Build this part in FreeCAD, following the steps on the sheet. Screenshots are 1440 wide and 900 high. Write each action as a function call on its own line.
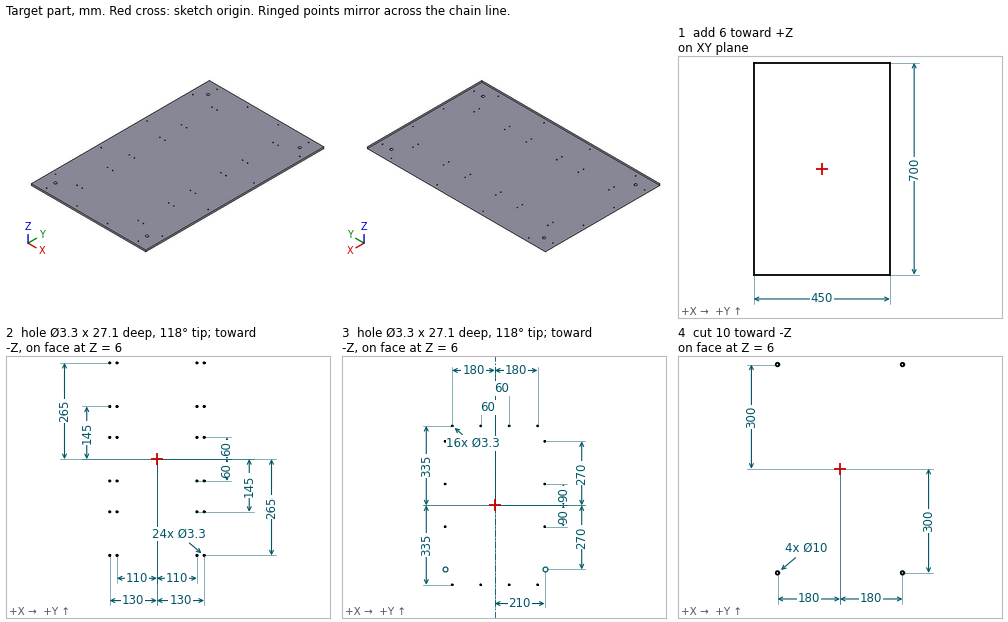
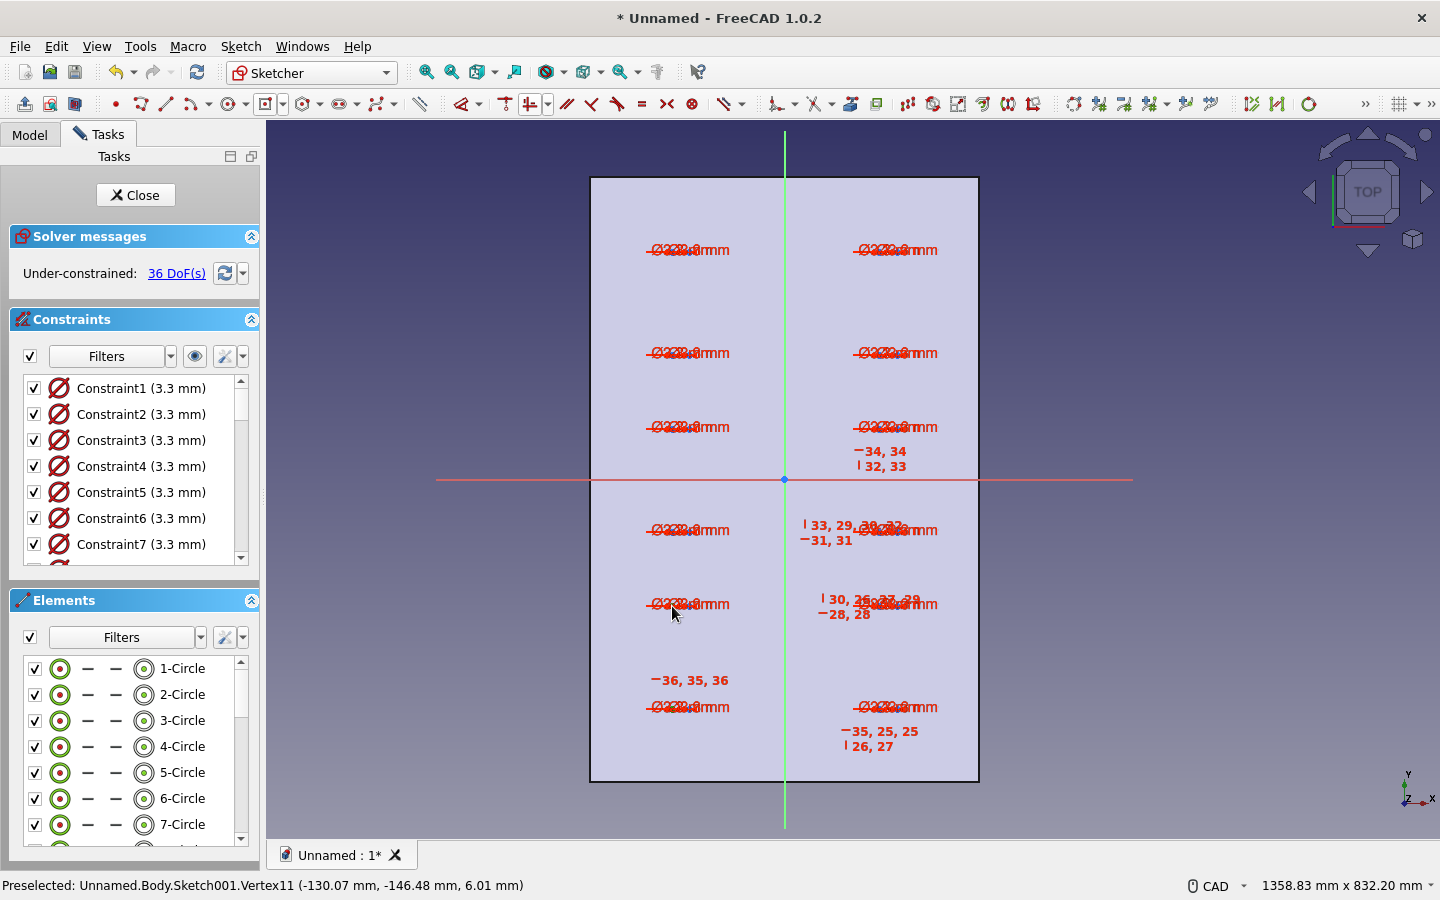
click(548, 104)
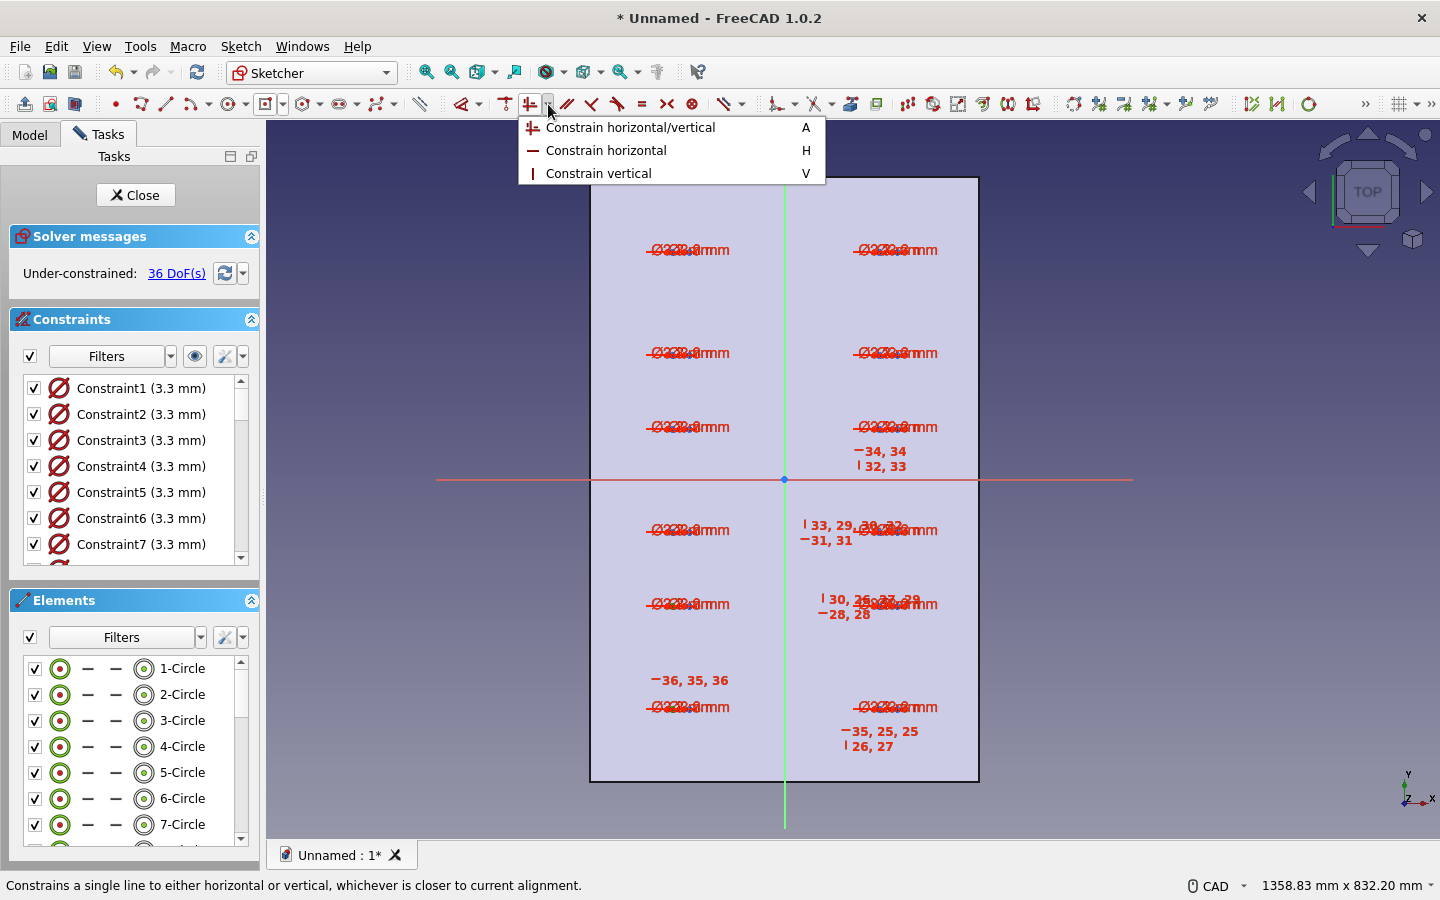
click(672, 174)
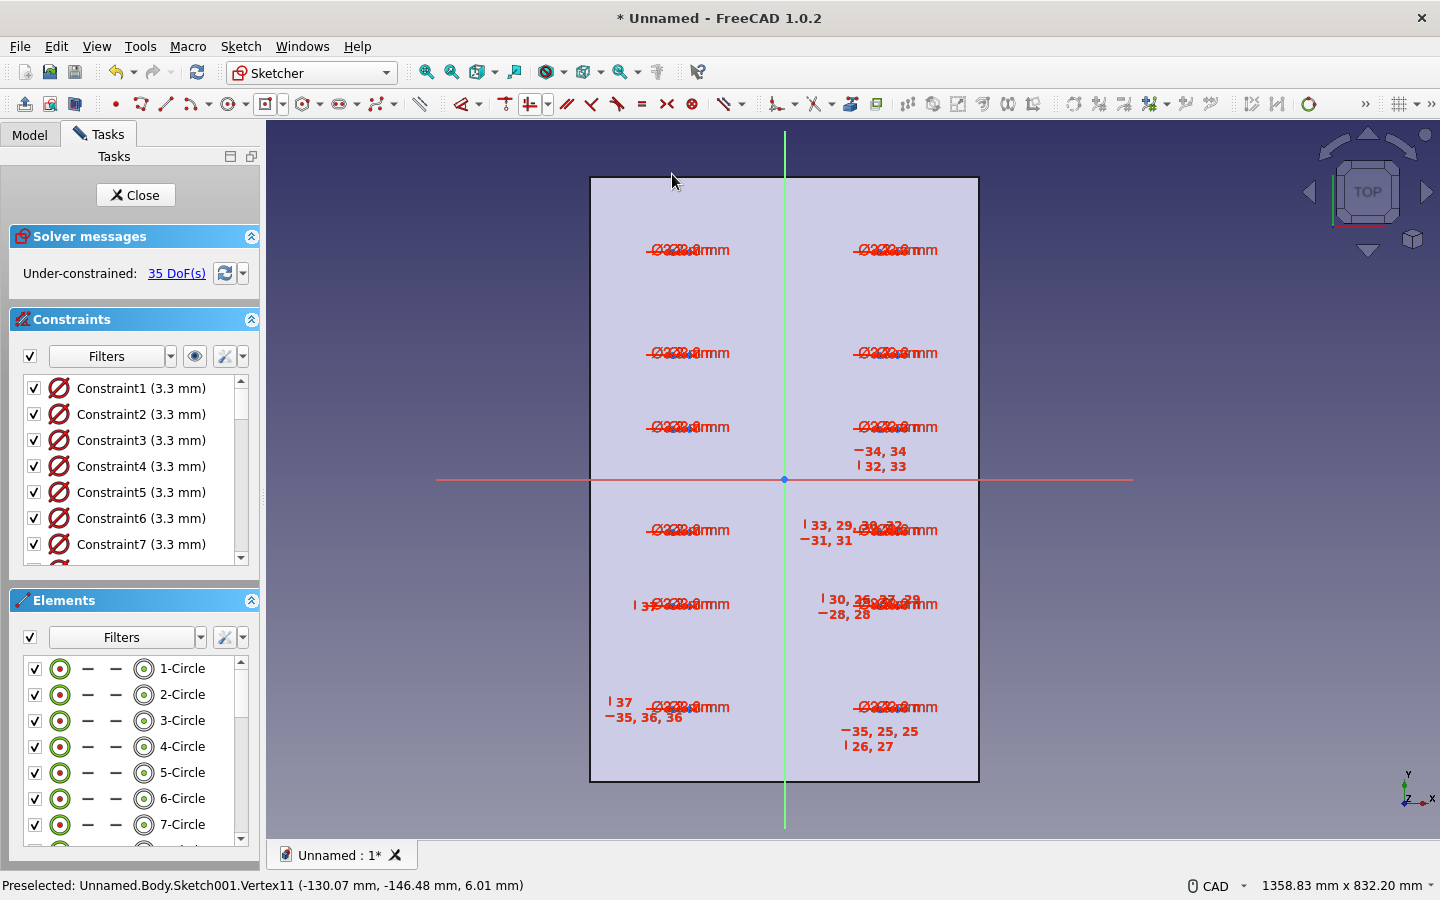
click(879, 606)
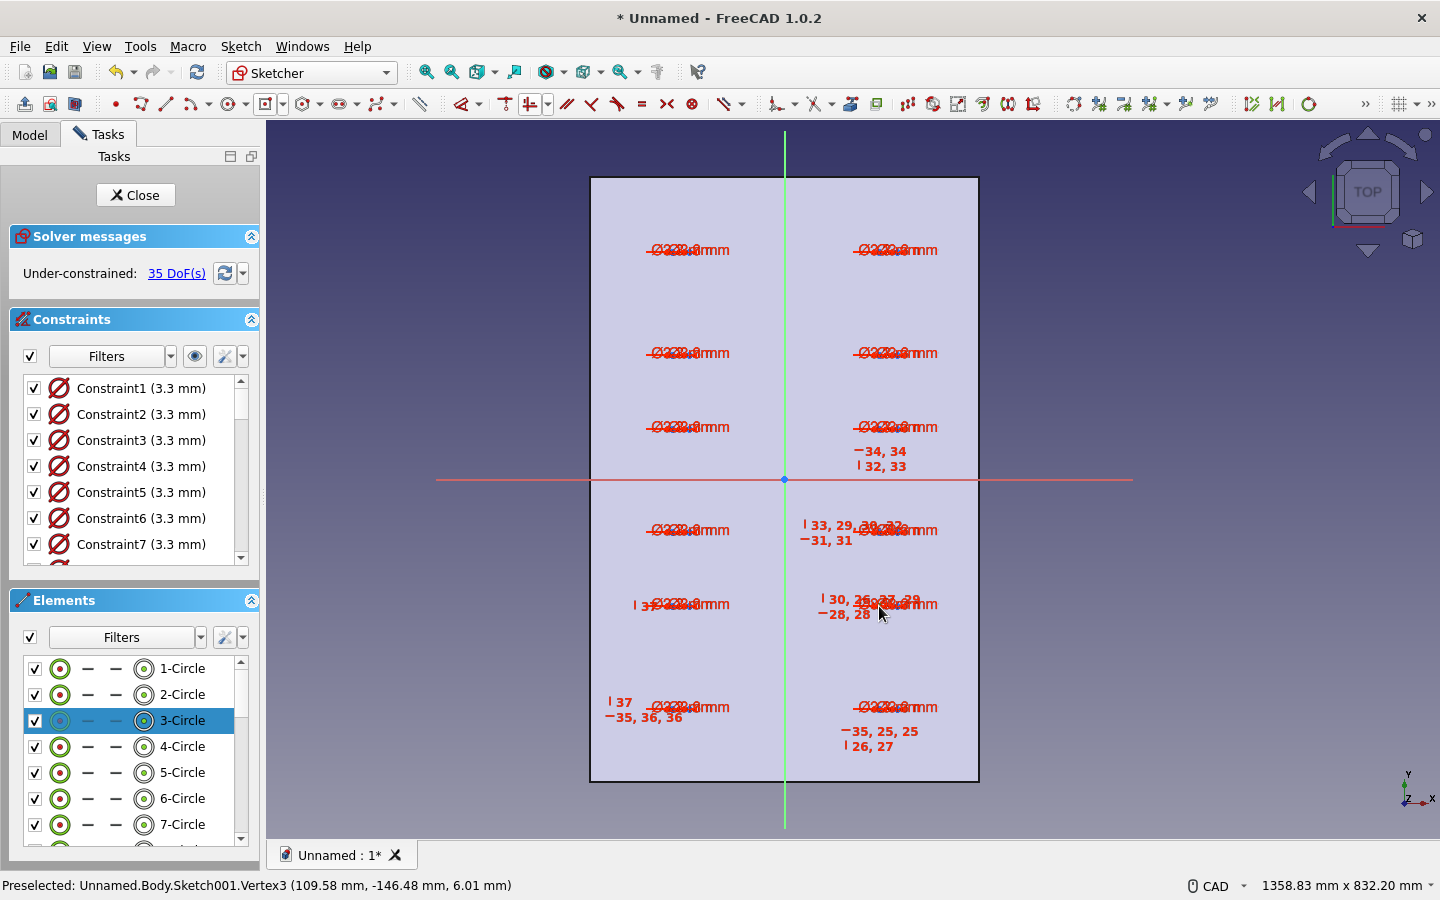
click(672, 606)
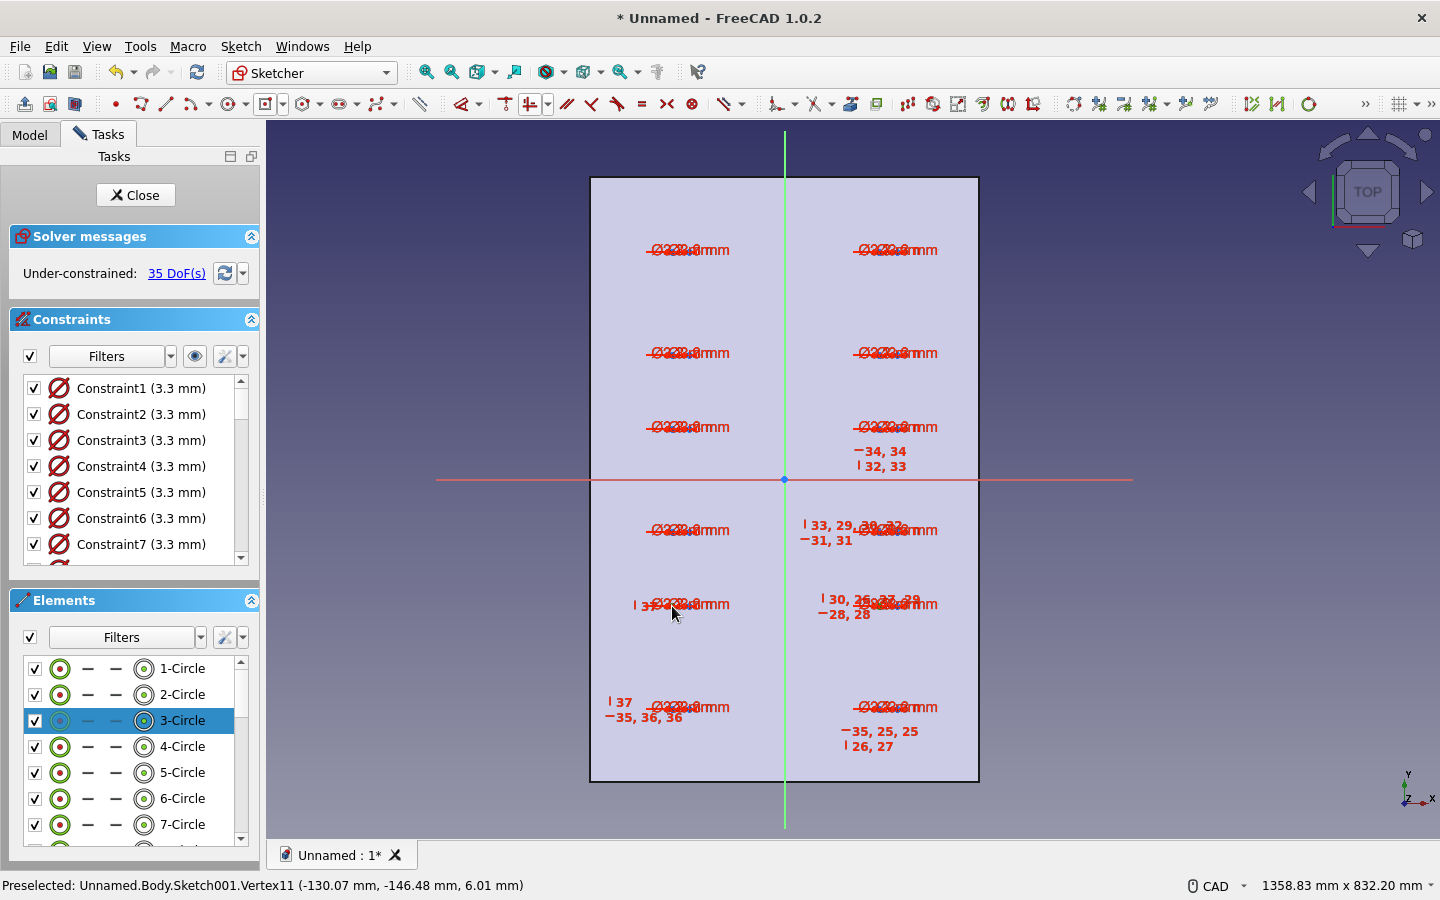
click(548, 104)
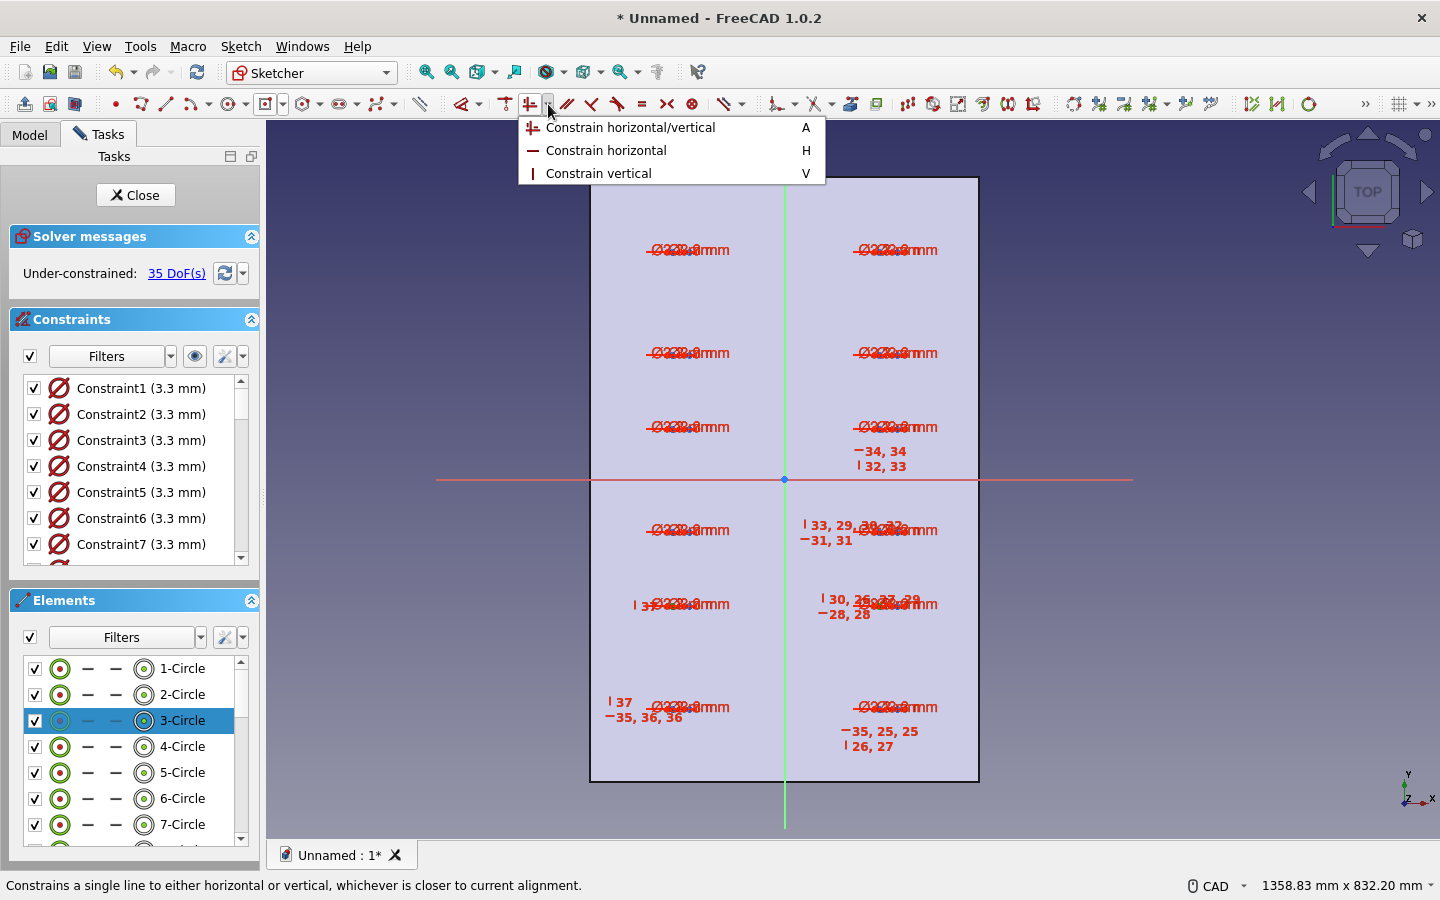
click(672, 150)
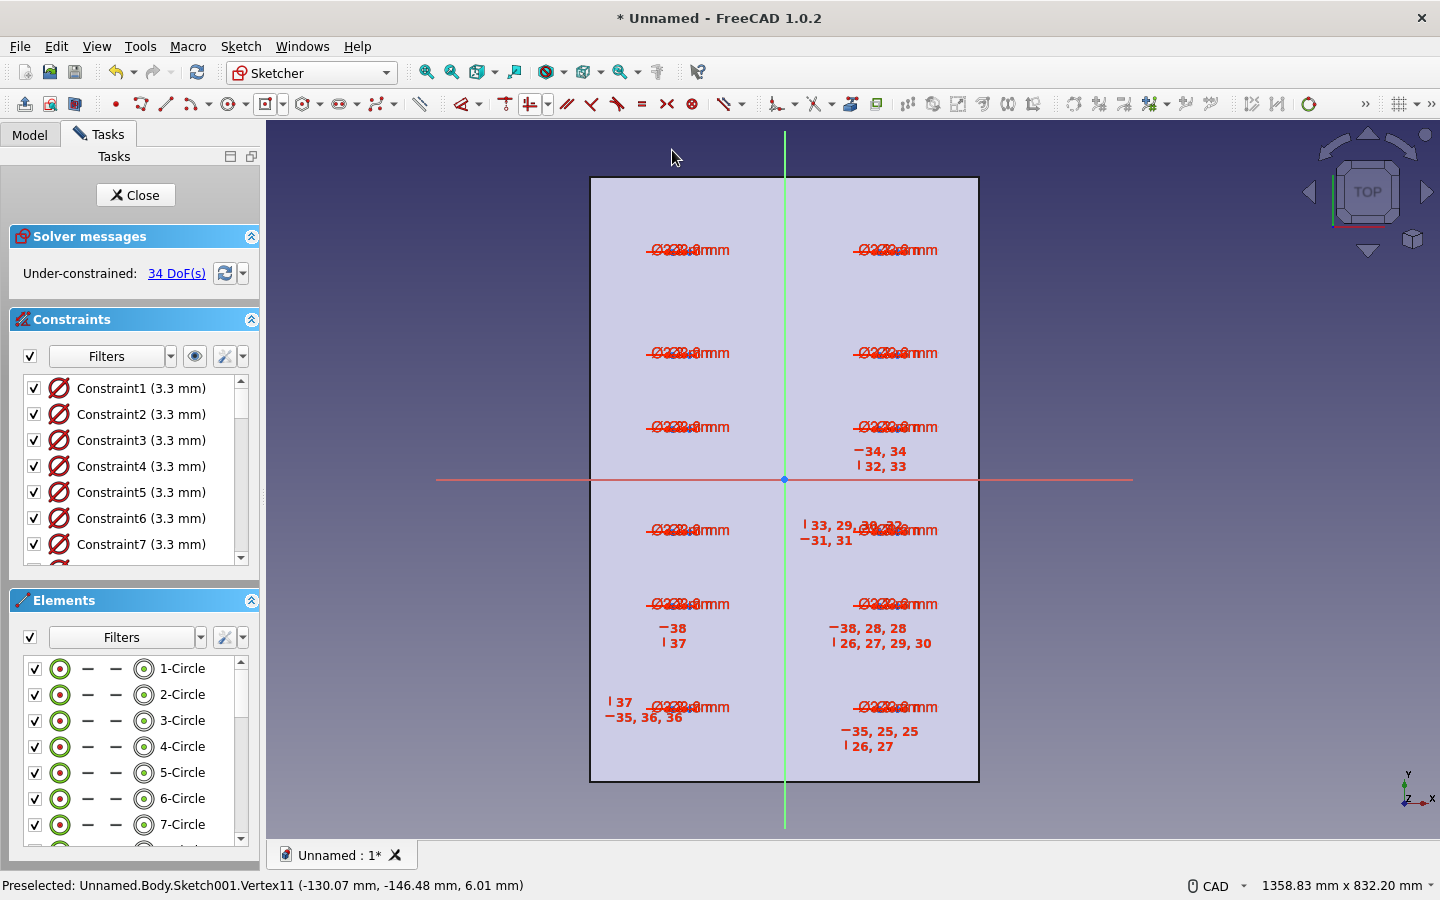
click(689, 709)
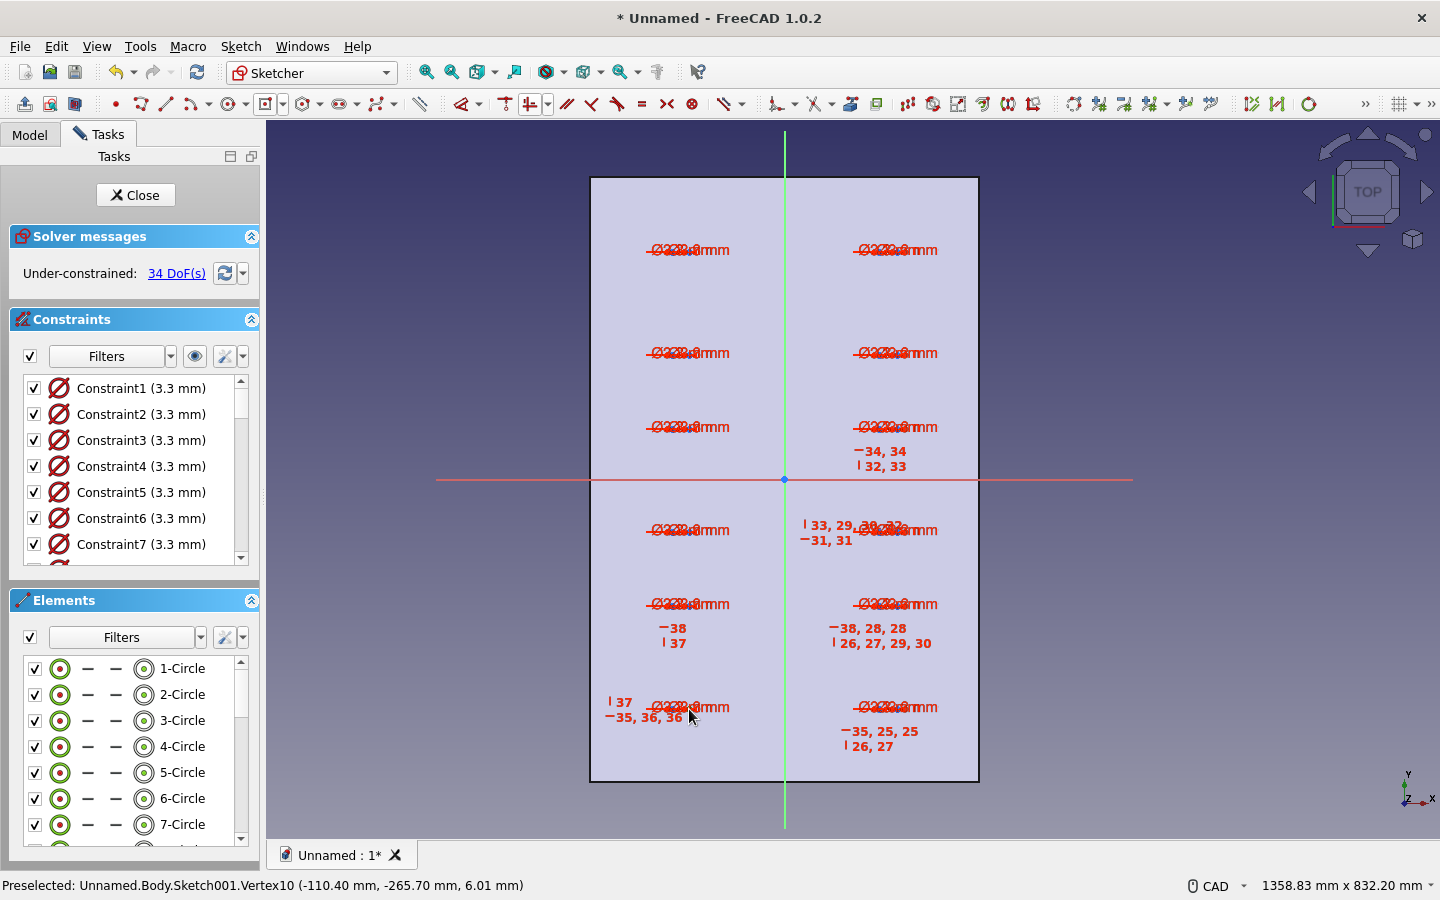
click(689, 606)